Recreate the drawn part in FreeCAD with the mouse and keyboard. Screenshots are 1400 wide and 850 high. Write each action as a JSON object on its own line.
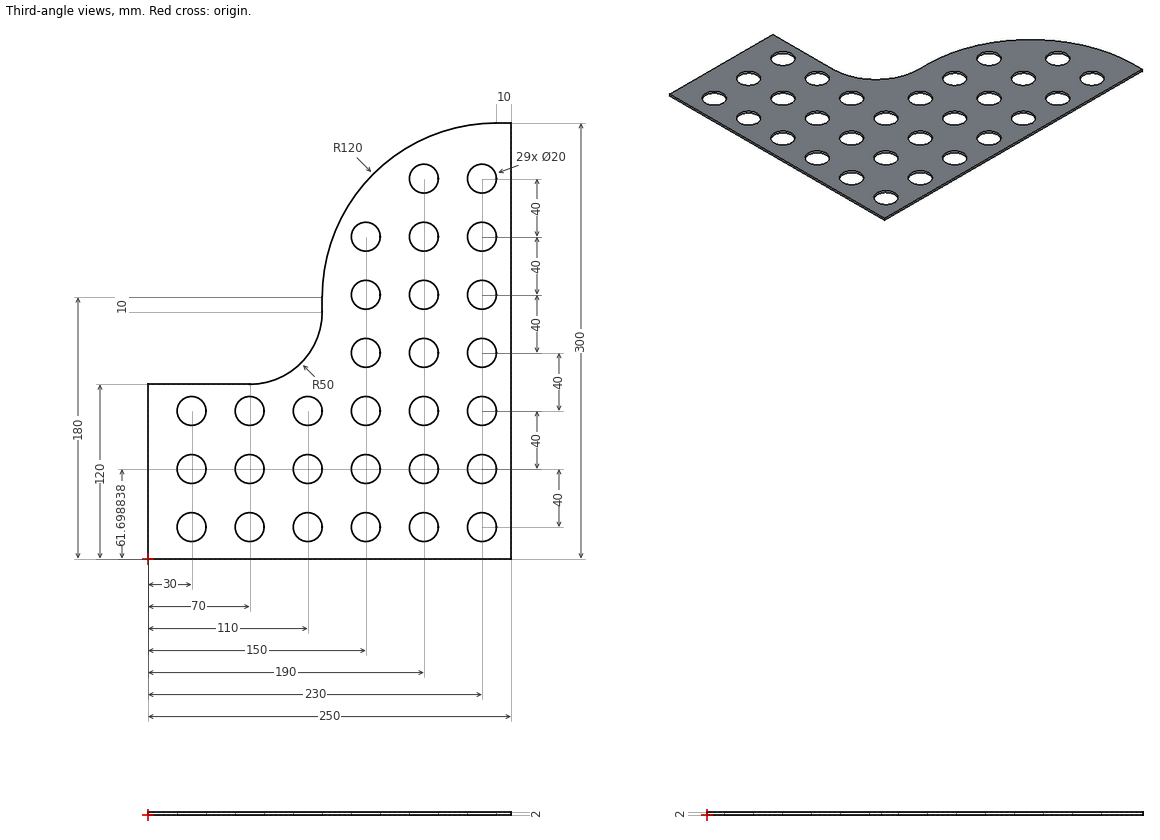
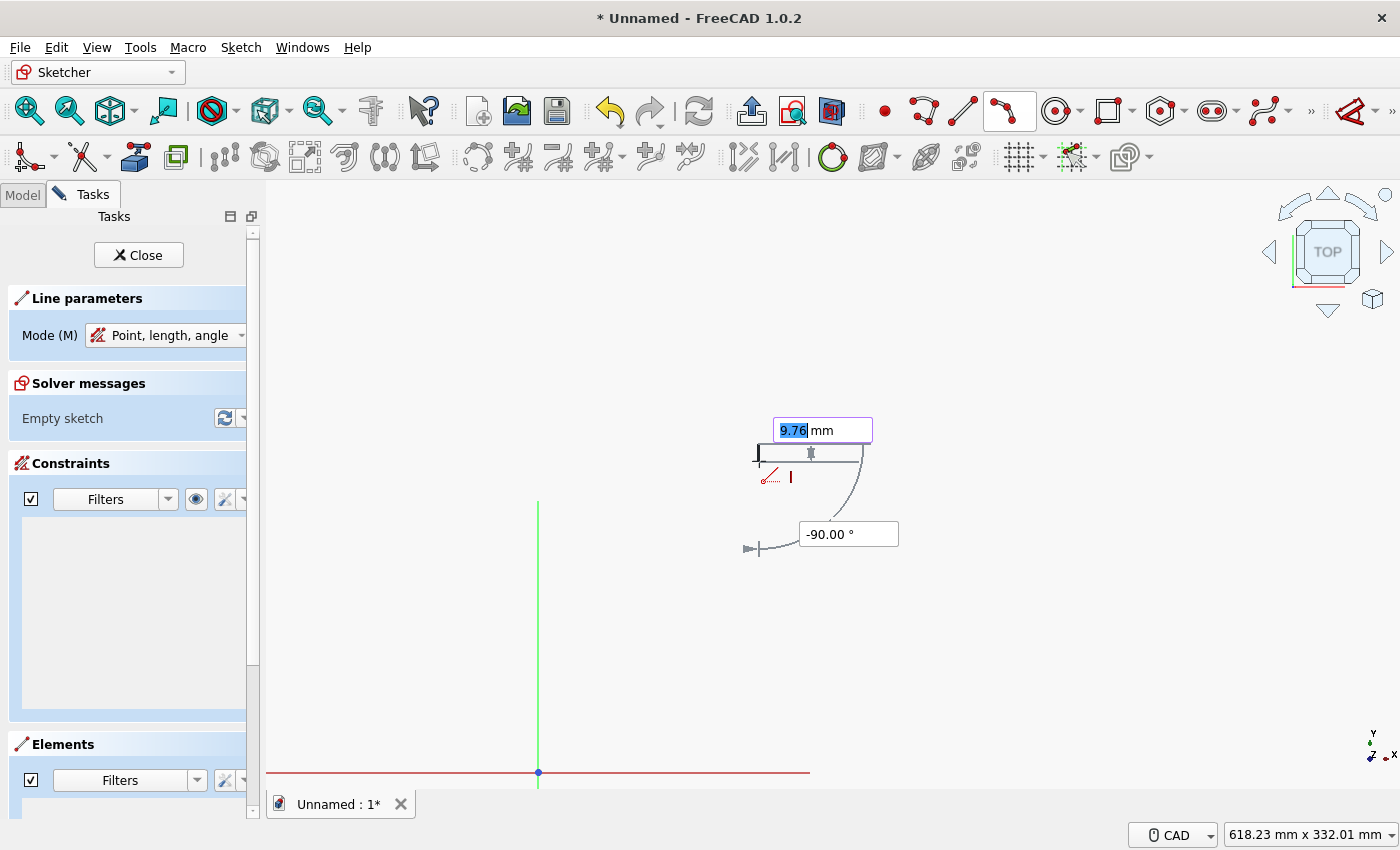
{"action": "left_click", "coordinate": [759, 461]}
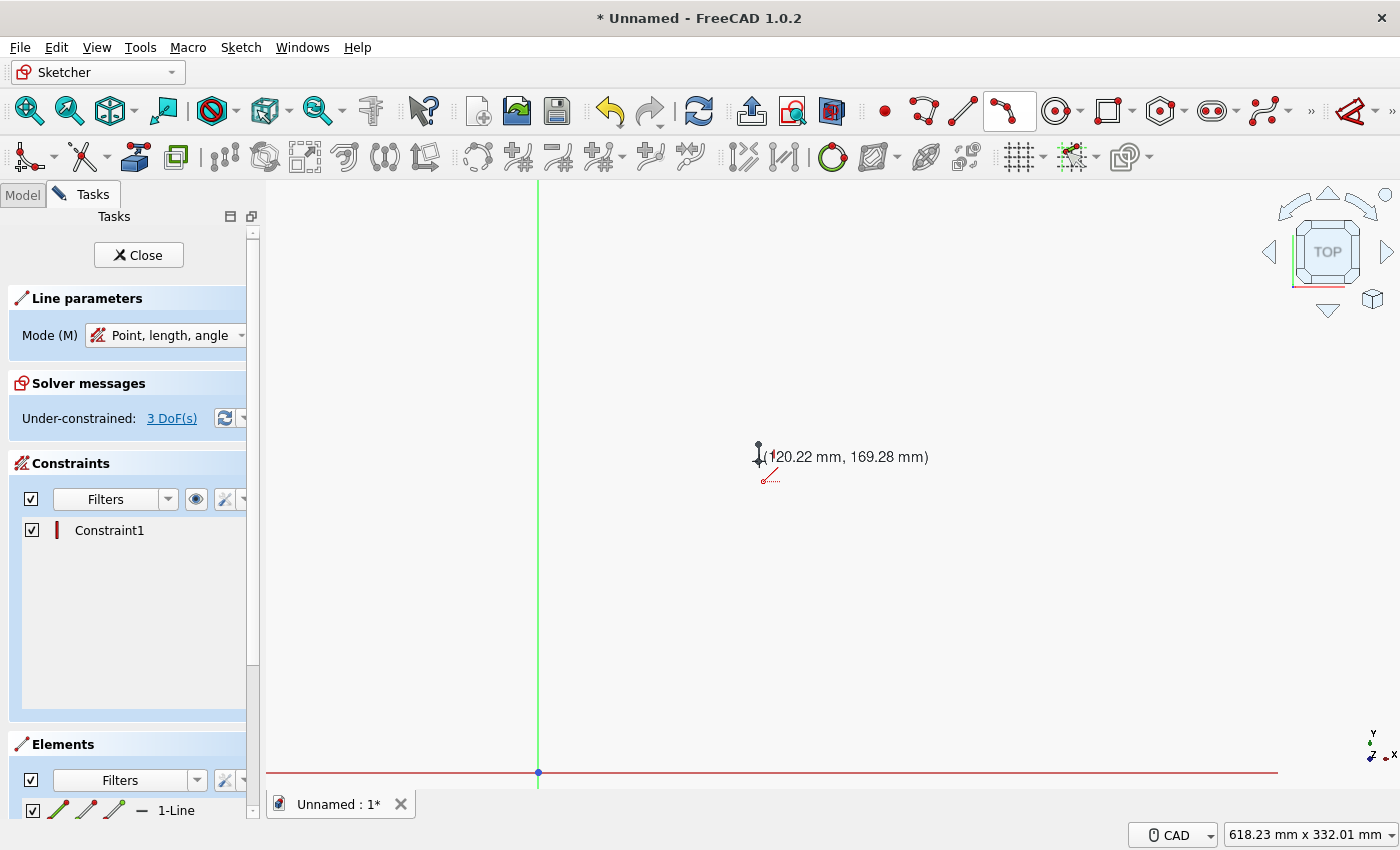
{"action": "left_click", "coordinate": [924, 112]}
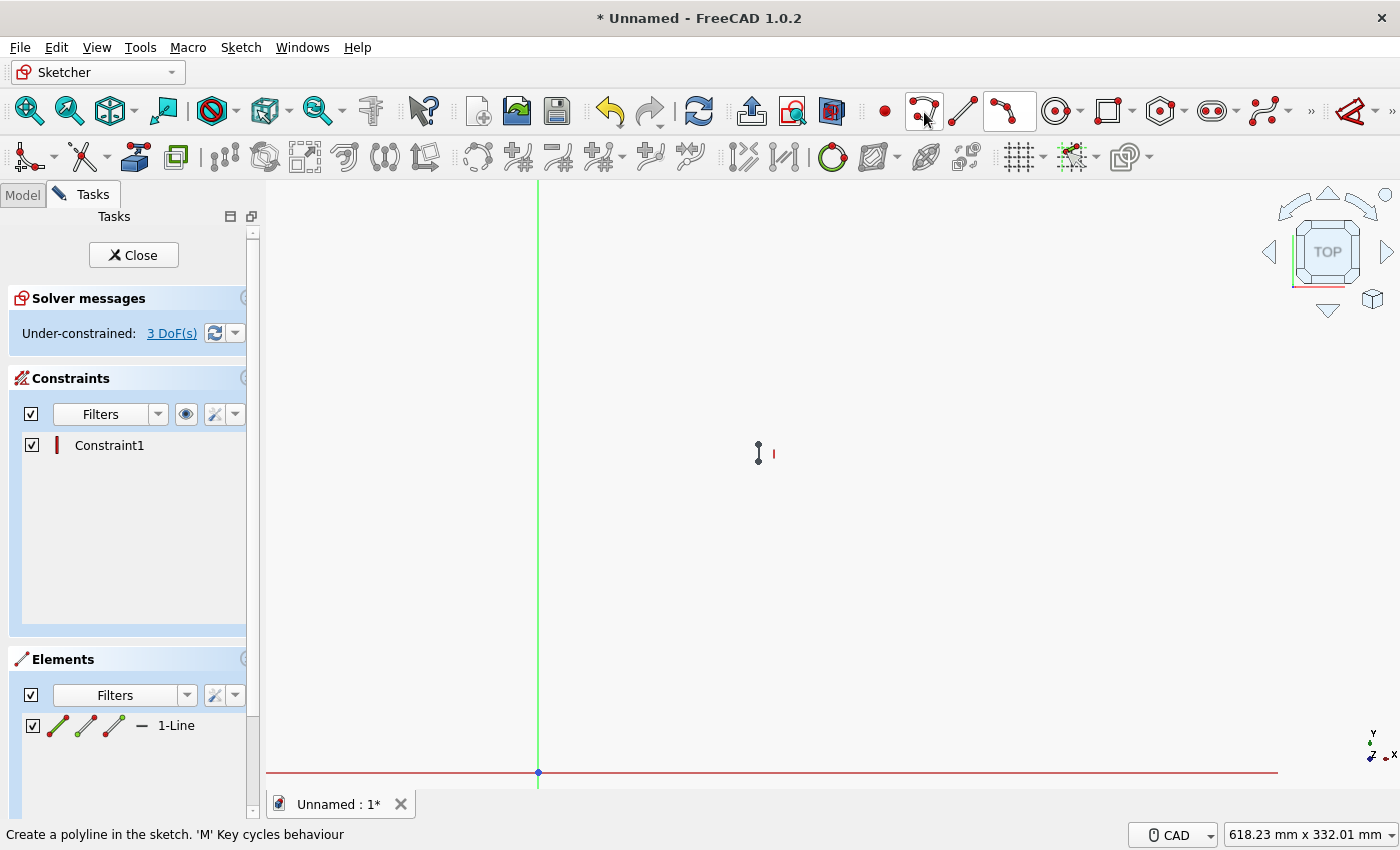
{"action": "left_click", "coordinate": [667, 552]}
{"action": "left_click", "coordinate": [538, 552]}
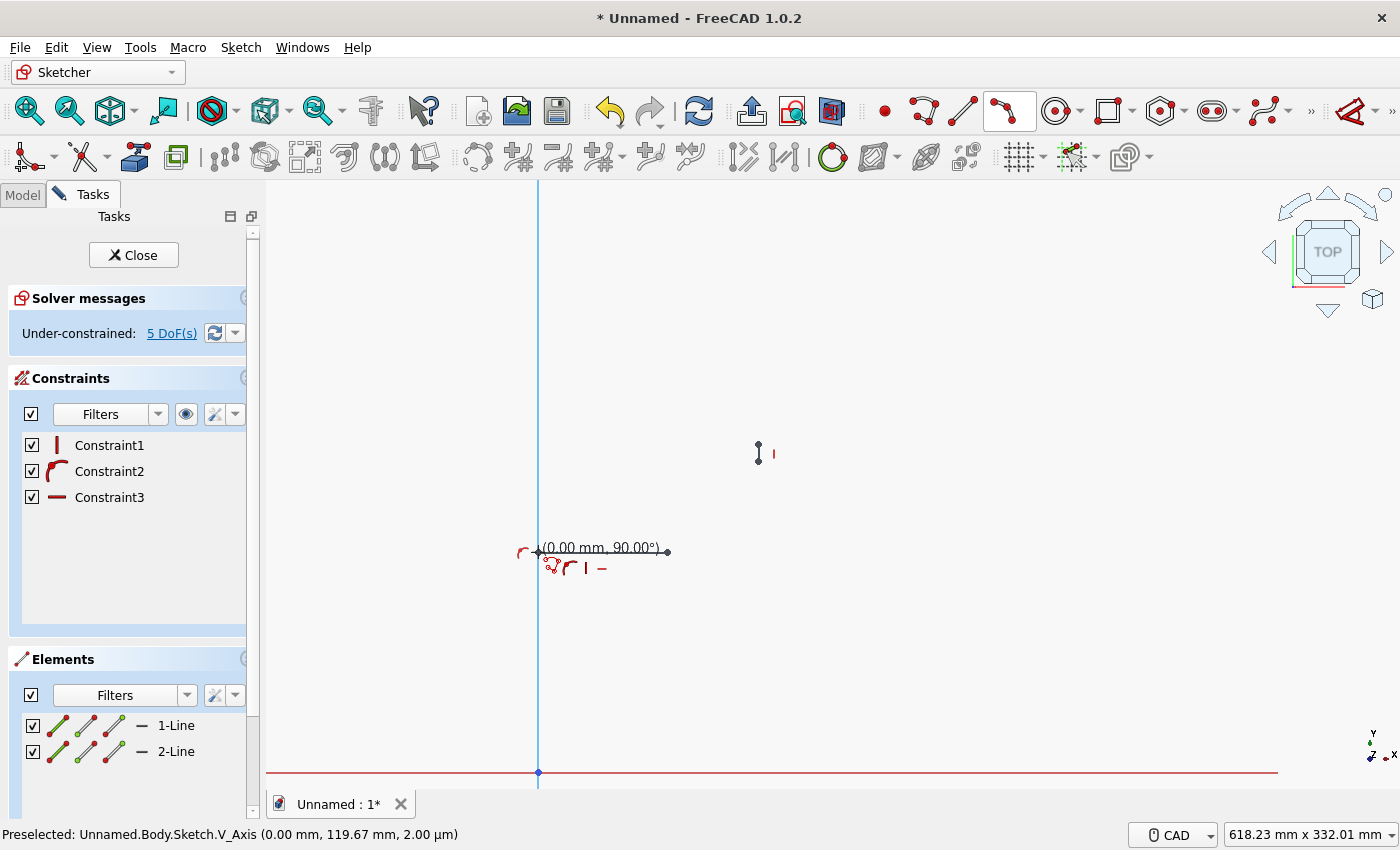
{"action": "scroll", "coordinate": [758, 458], "scroll_direction": "down", "scroll_amount": 2}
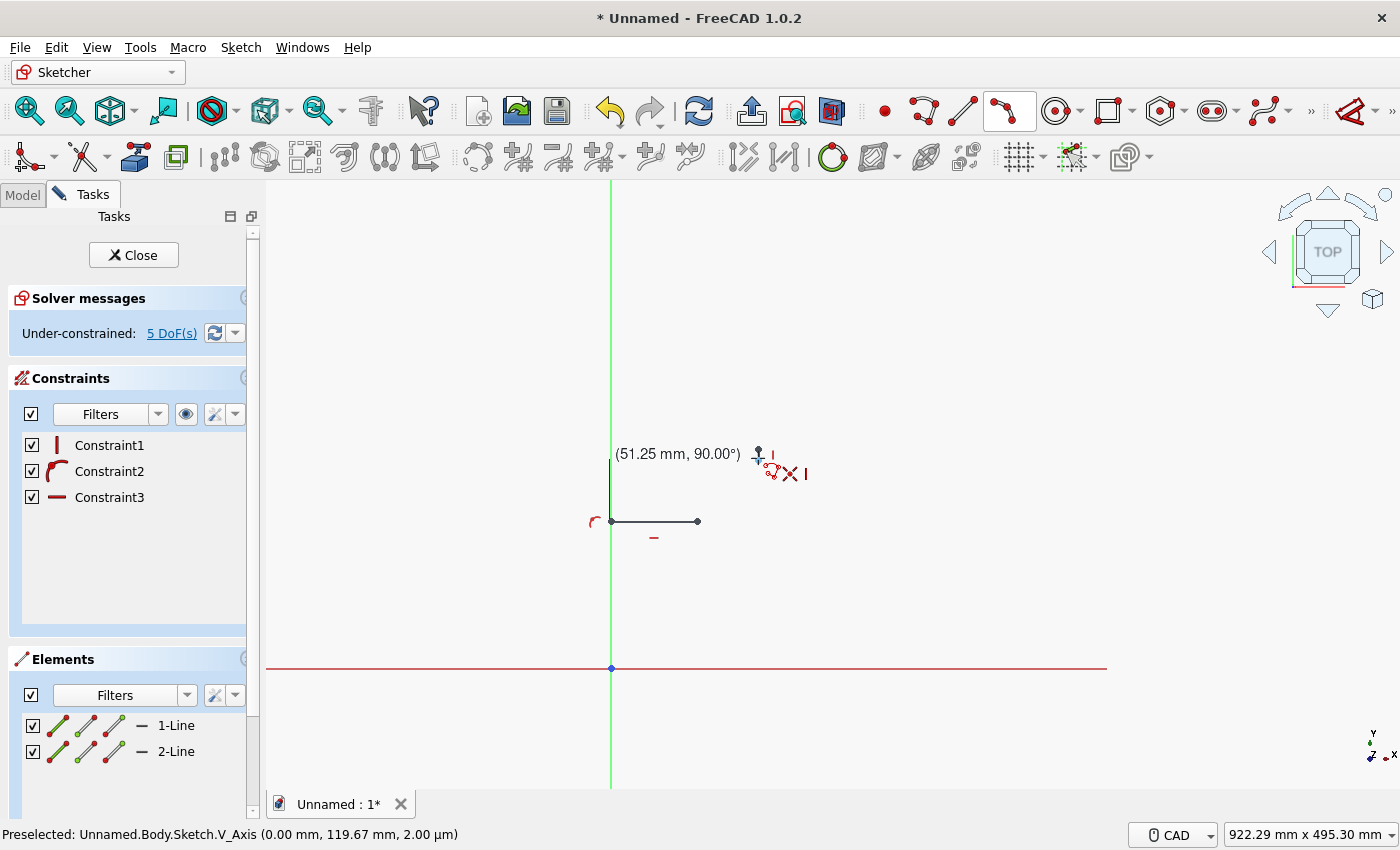
{"action": "left_click", "coordinate": [611, 669]}
{"action": "left_click", "coordinate": [918, 660]}
{"action": "left_click", "coordinate": [918, 300]}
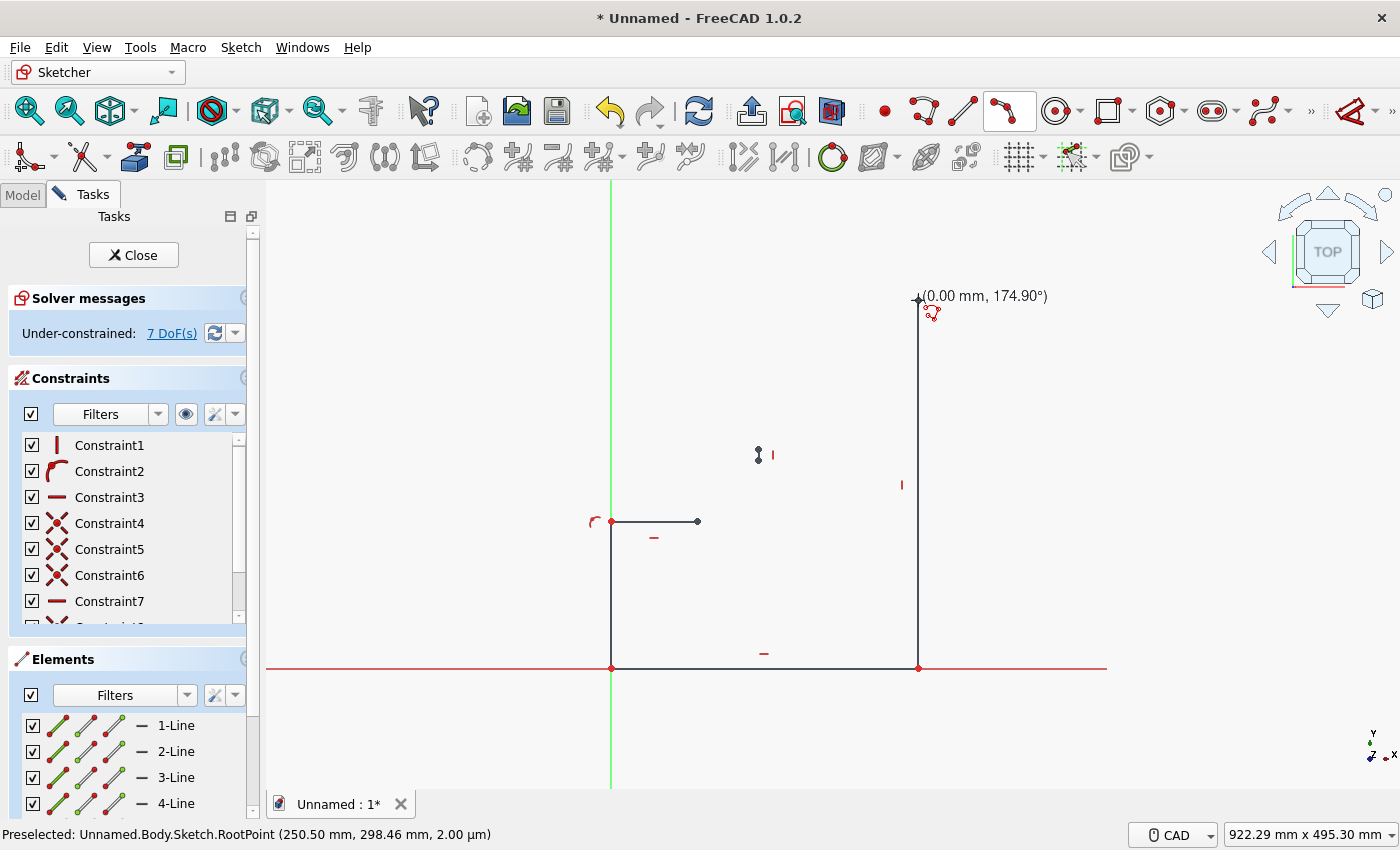
{"action": "scroll", "coordinate": [906, 300], "scroll_direction": "up", "scroll_amount": 2}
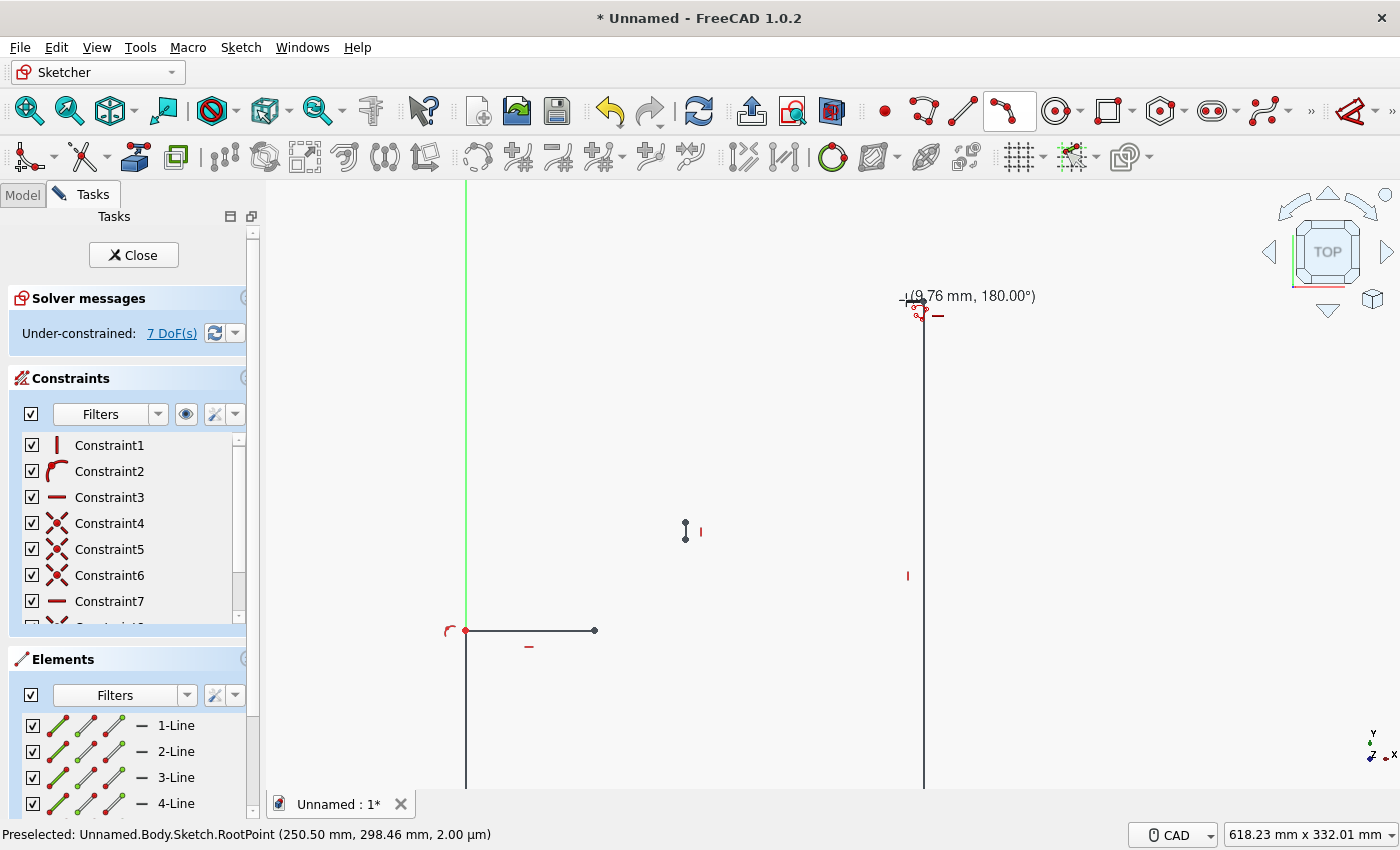
{"action": "left_click", "coordinate": [906, 300]}
{"action": "right_click", "coordinate": [906, 300]}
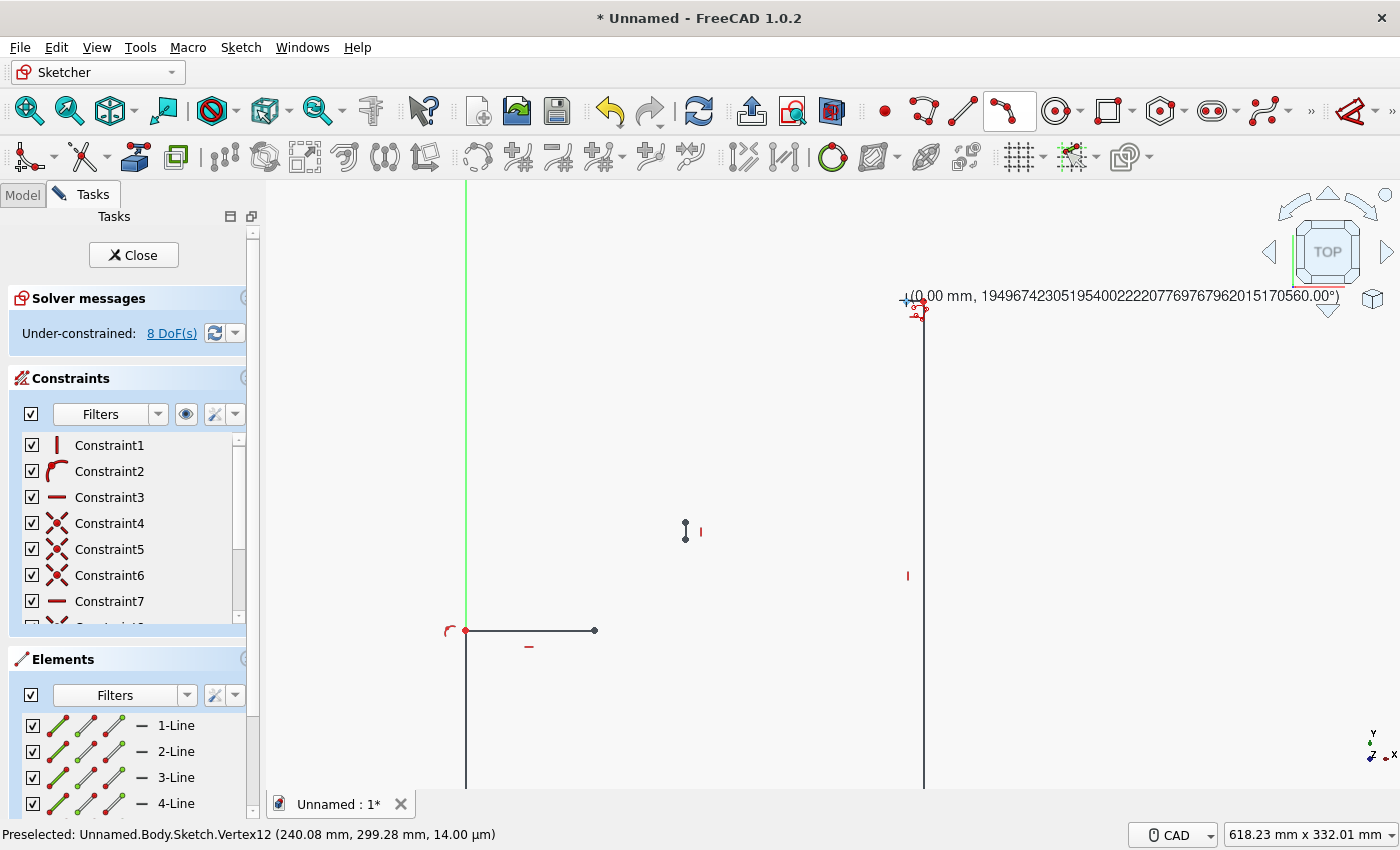
{"action": "left_click", "coordinate": [1004, 112]}